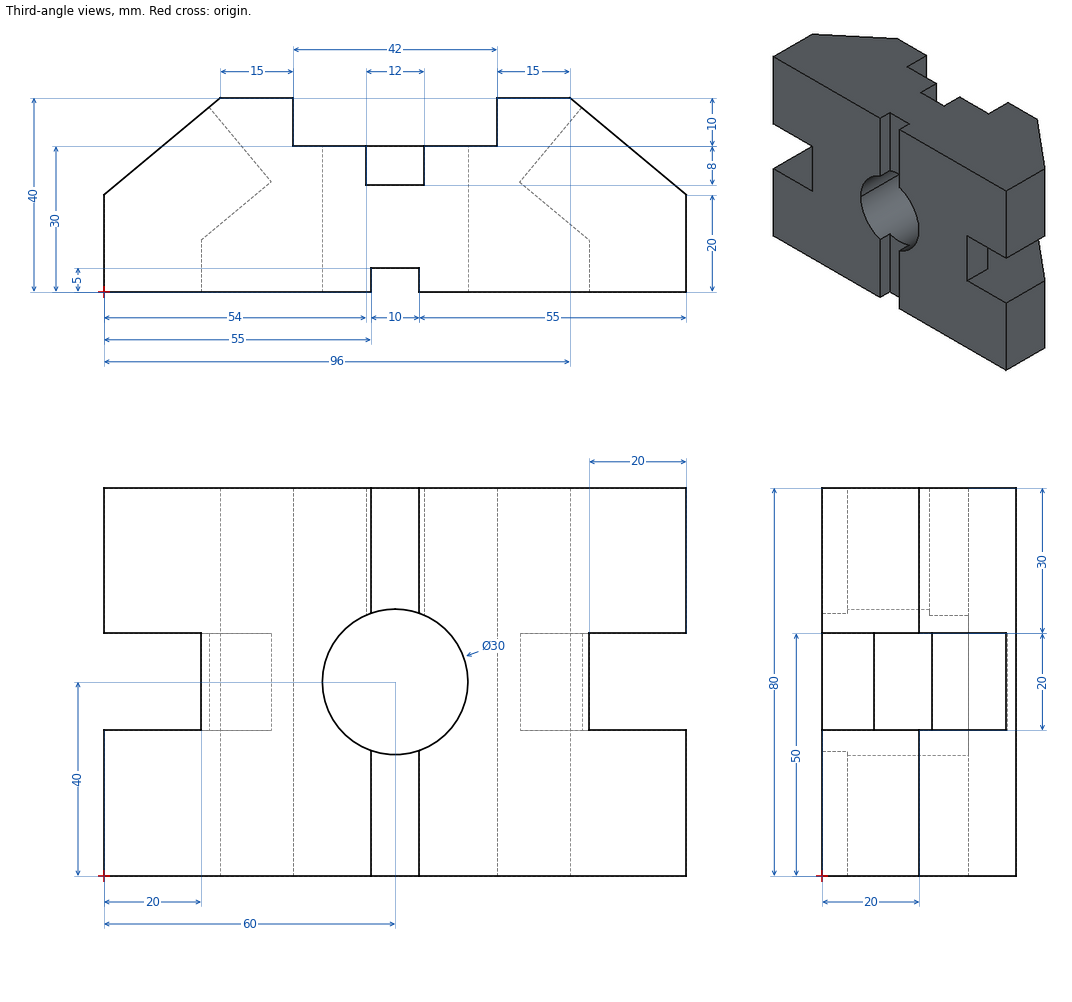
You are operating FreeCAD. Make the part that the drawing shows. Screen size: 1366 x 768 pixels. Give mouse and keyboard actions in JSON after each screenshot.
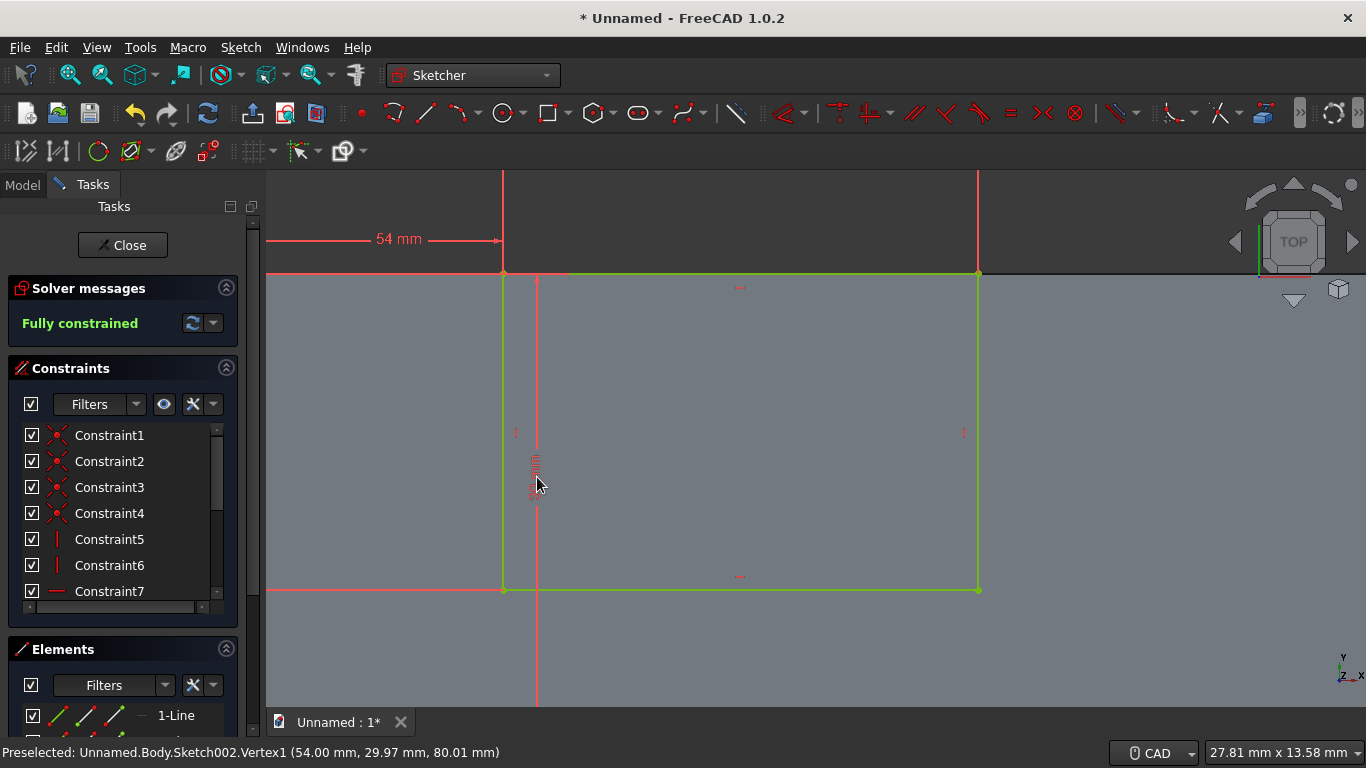
{"action": "left_click", "coordinate": [123, 245]}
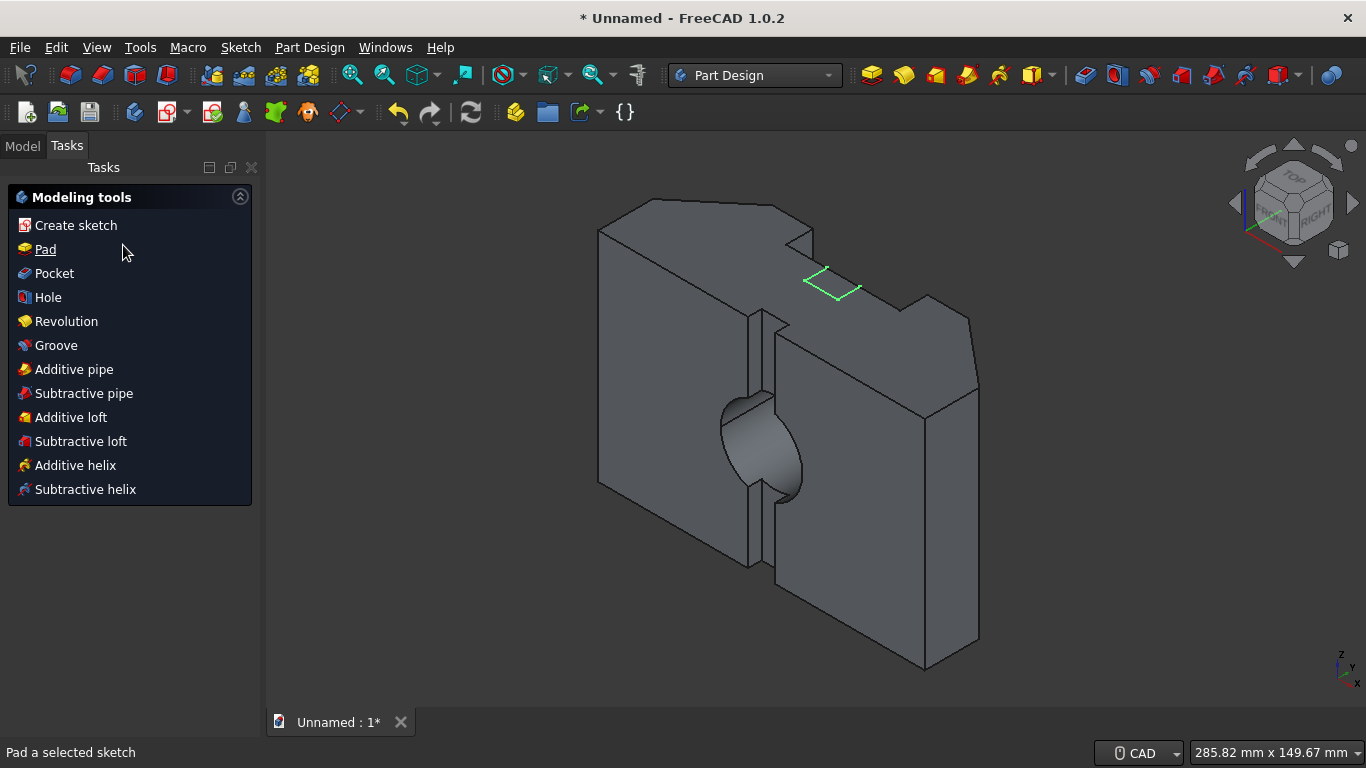
{"action": "left_click", "coordinate": [1086, 76]}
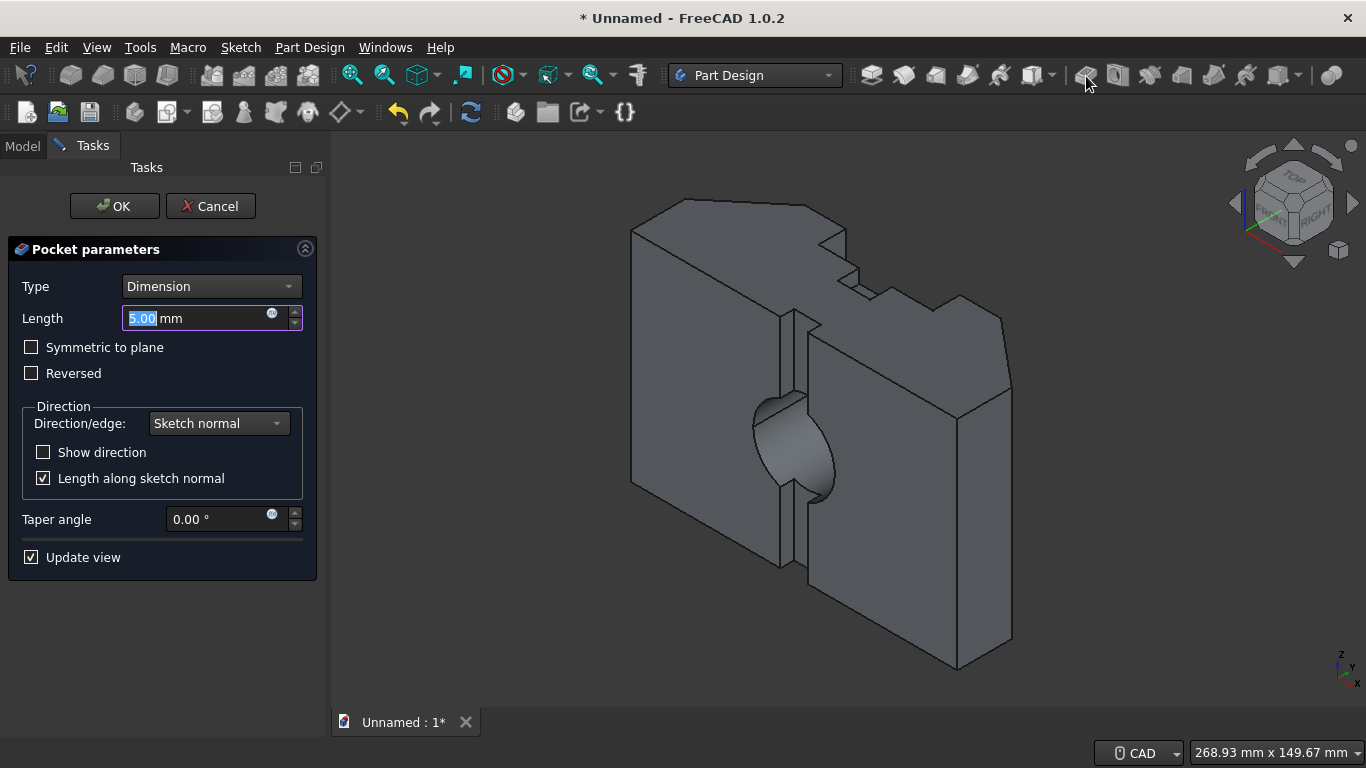
{"action": "type", "text": "30"}
{"action": "key", "text": "Tab"}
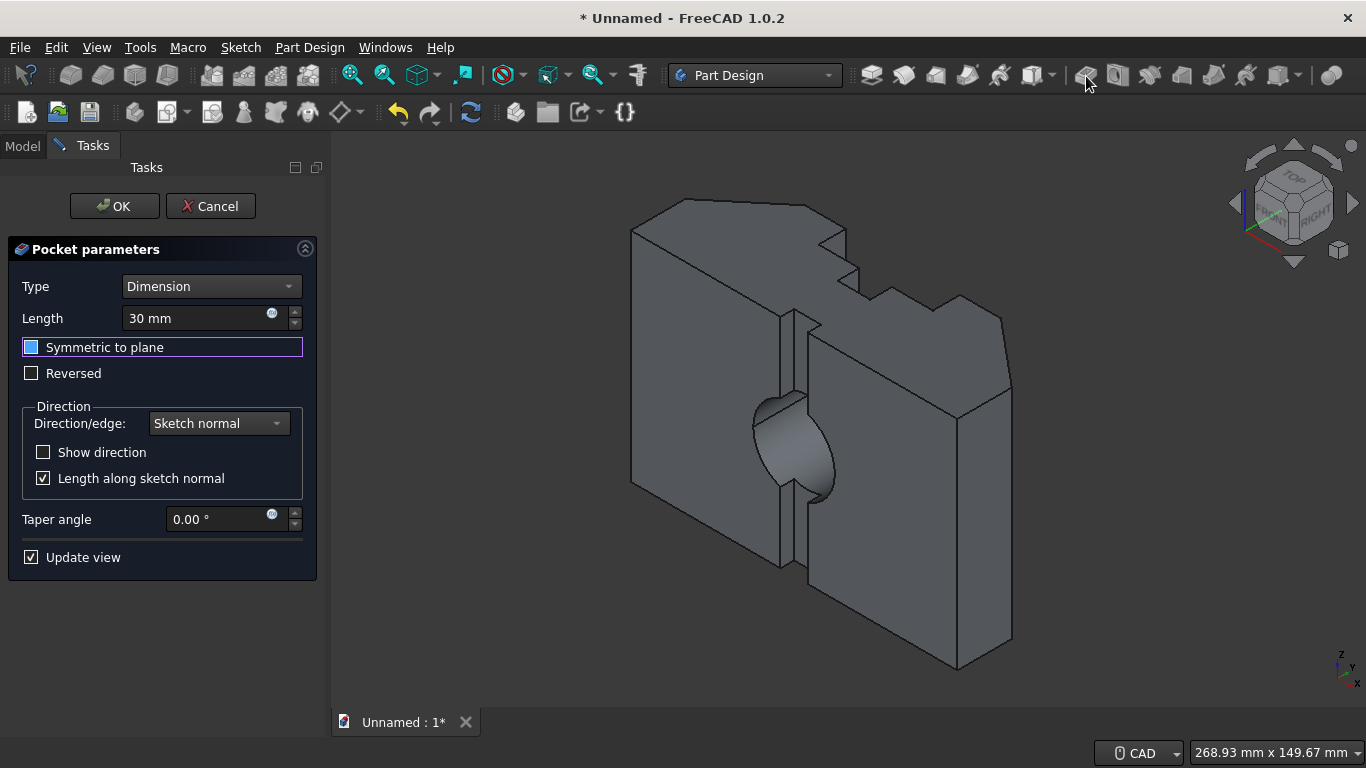
{"action": "left_click", "coordinate": [115, 206]}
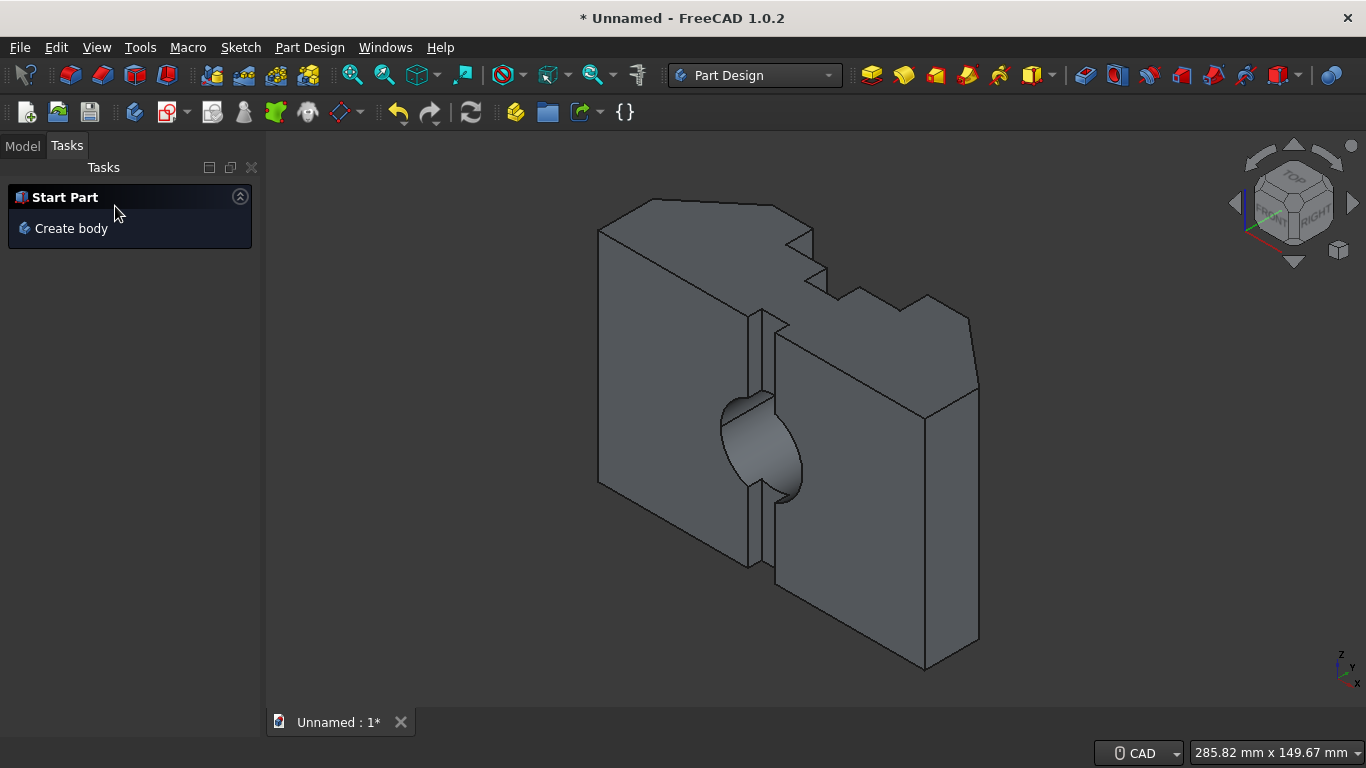
{"action": "left_click", "coordinate": [952, 456]}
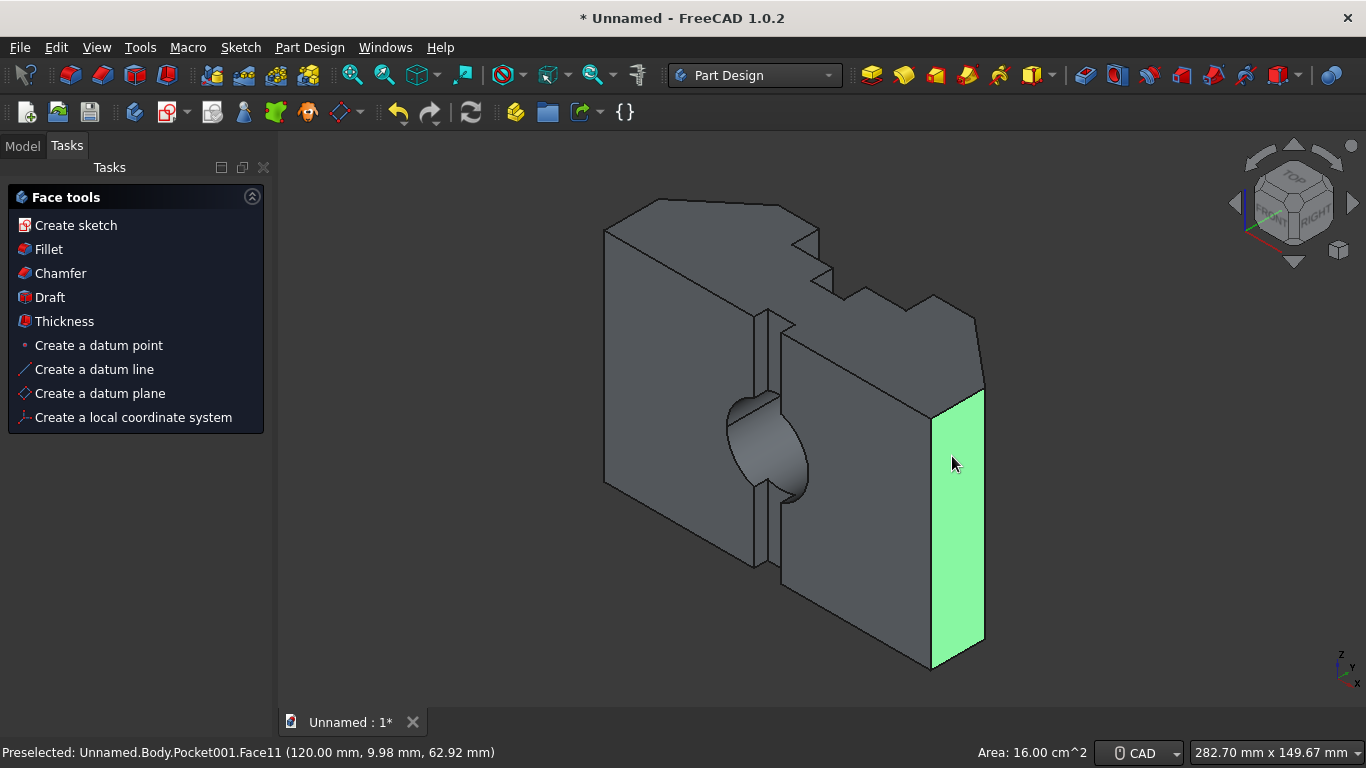
{"action": "left_click", "coordinate": [168, 112]}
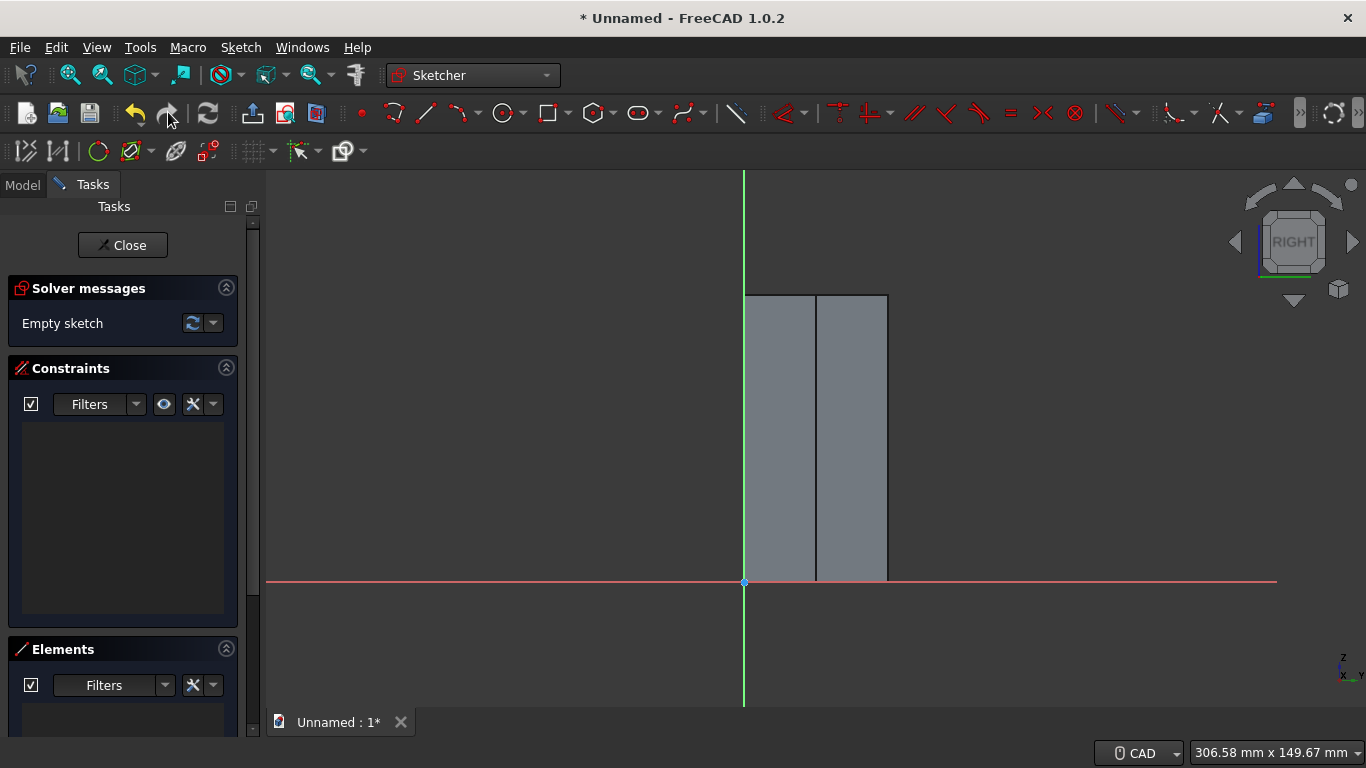
{"action": "scroll", "coordinate": [788, 439], "scroll_direction": "up", "scroll_amount": 8}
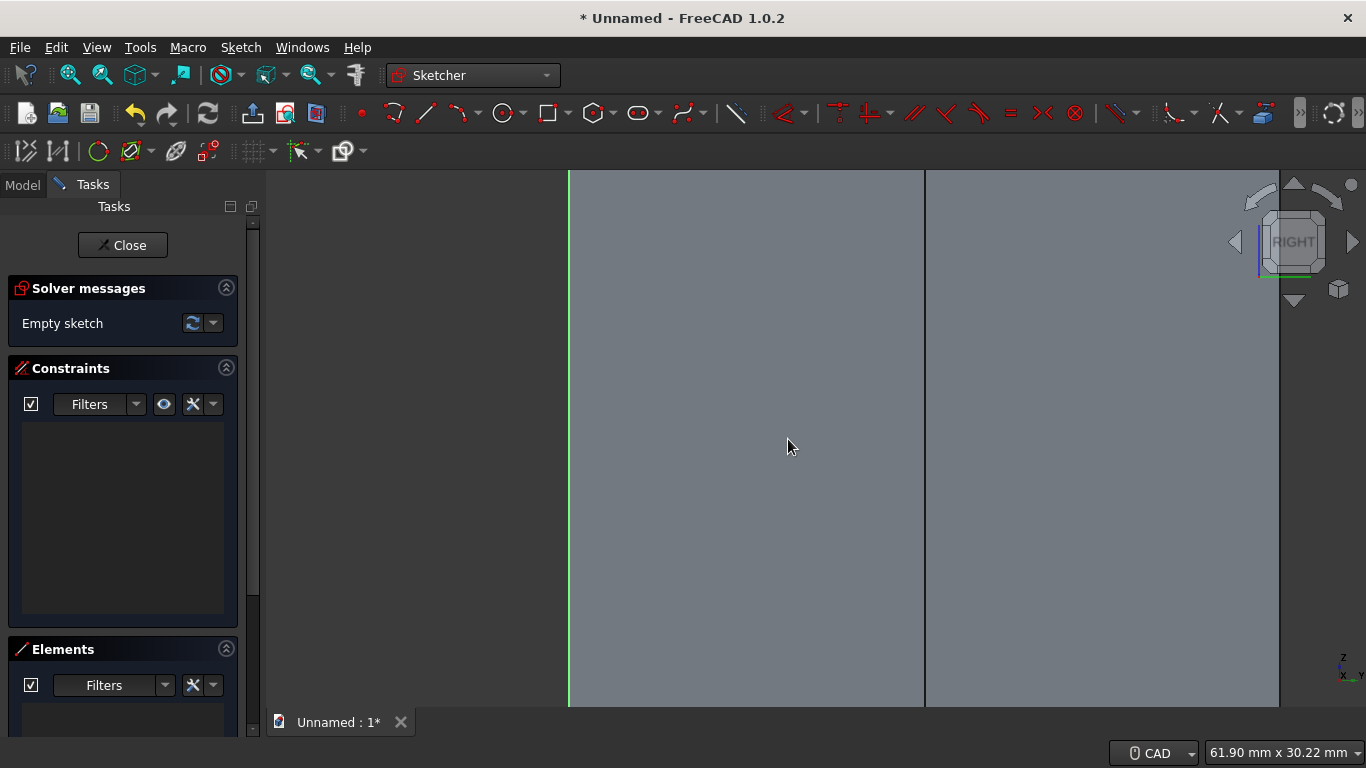
{"action": "left_click", "coordinate": [548, 114]}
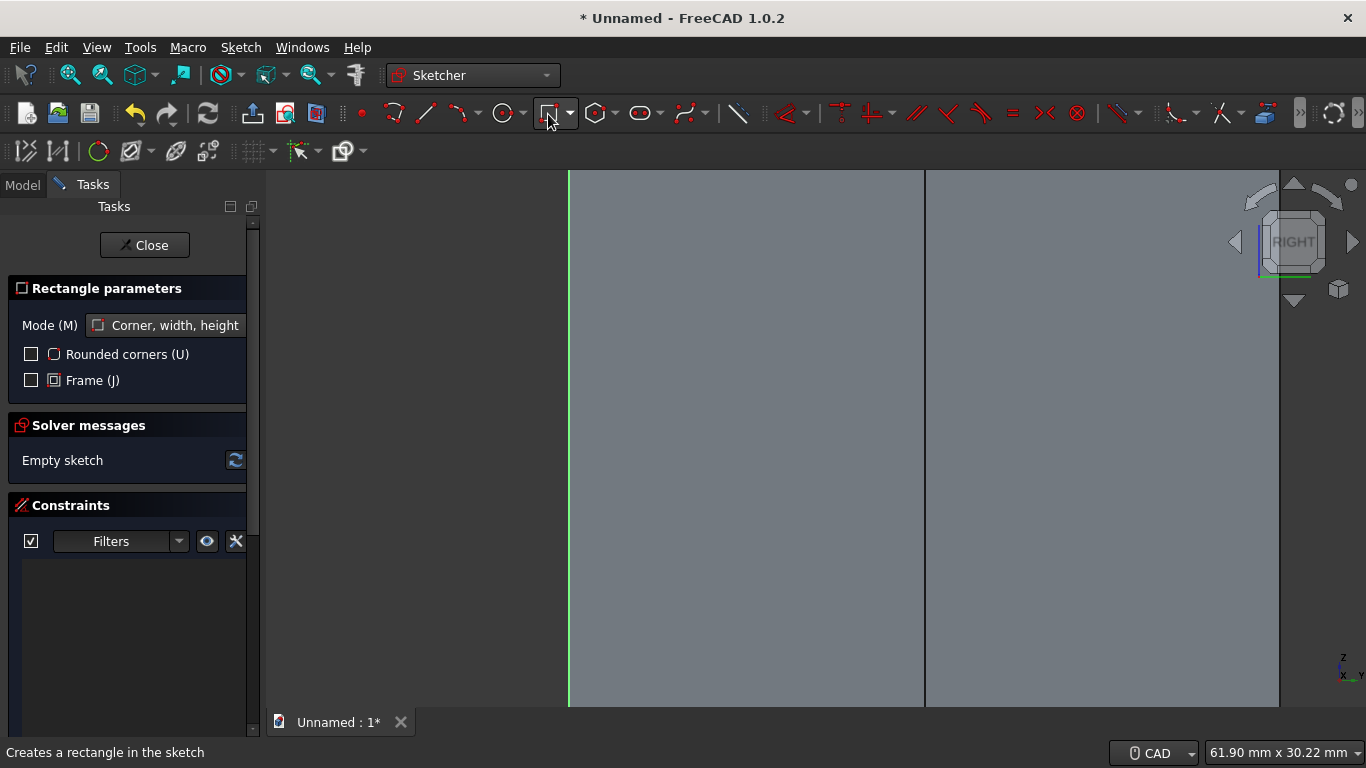
{"action": "left_click", "coordinate": [569, 257]}
{"action": "mouse_move", "coordinate": [925, 612]}